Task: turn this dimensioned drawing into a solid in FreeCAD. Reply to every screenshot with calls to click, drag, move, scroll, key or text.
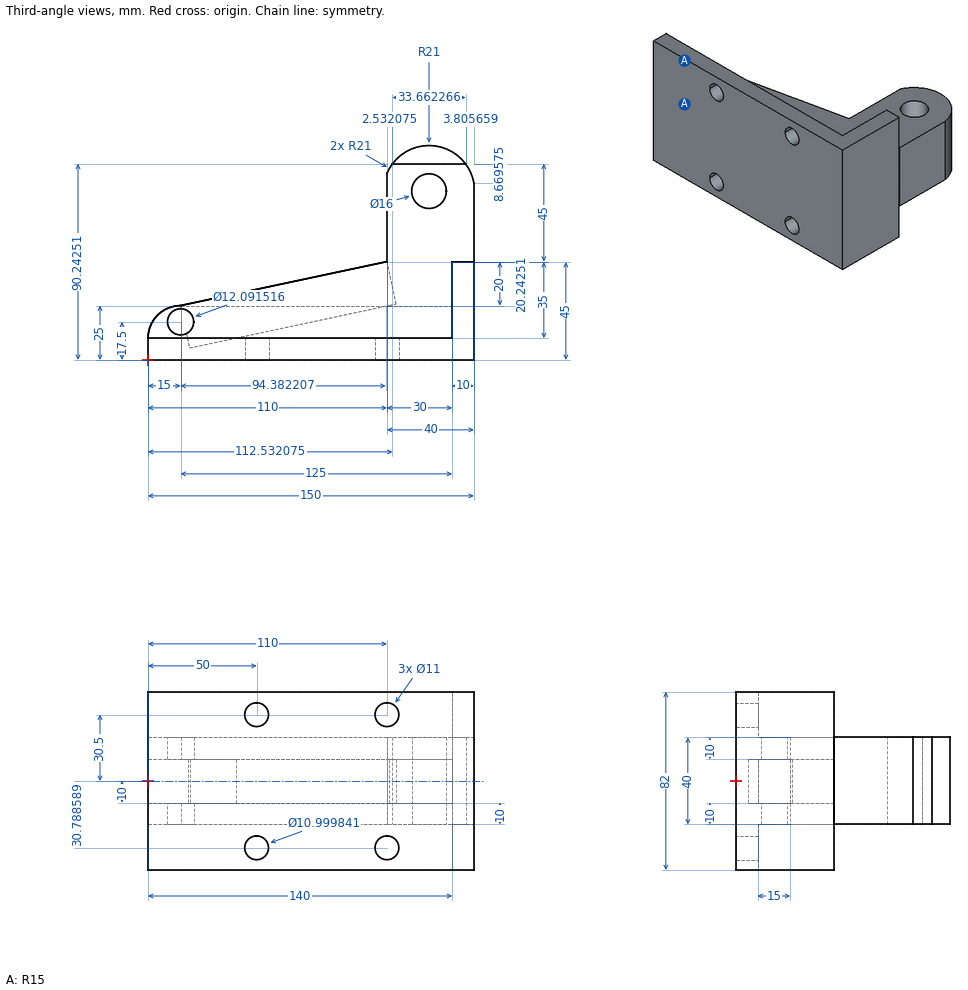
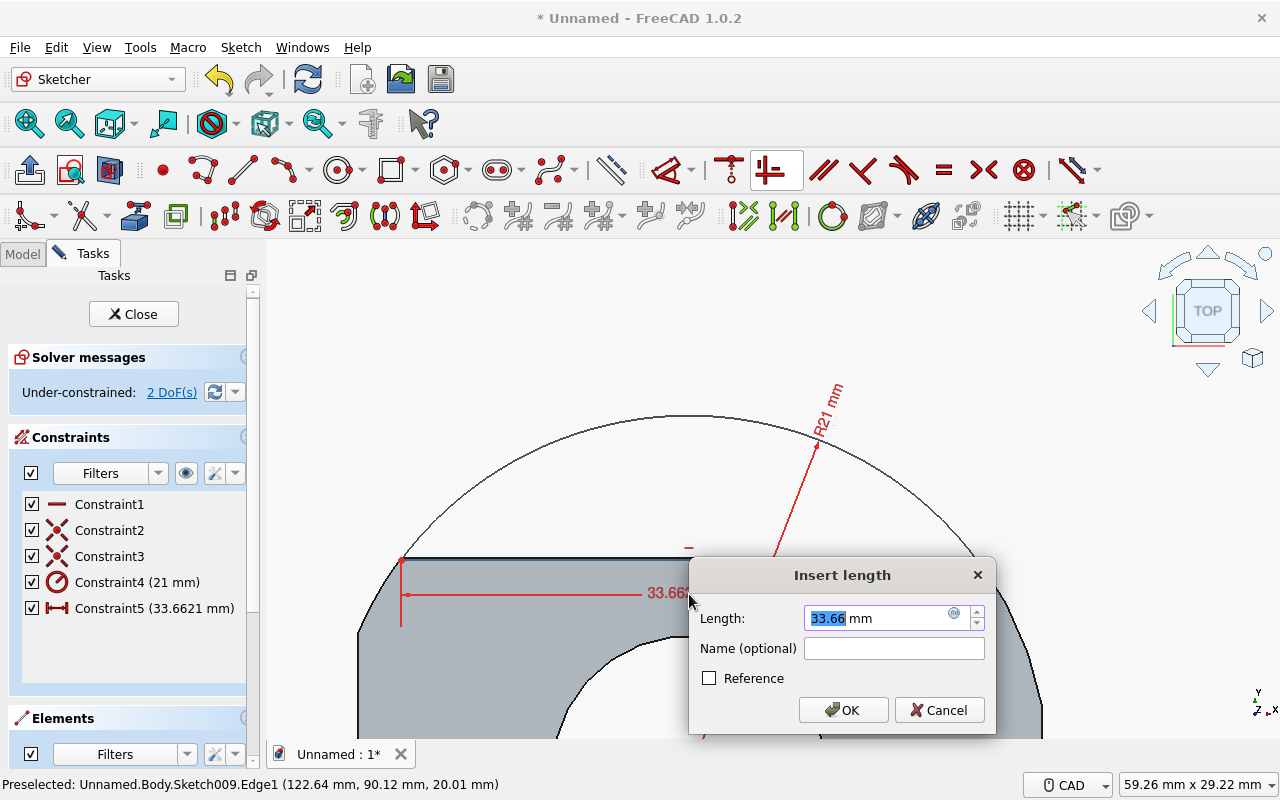
text(33.662266)
key(Return)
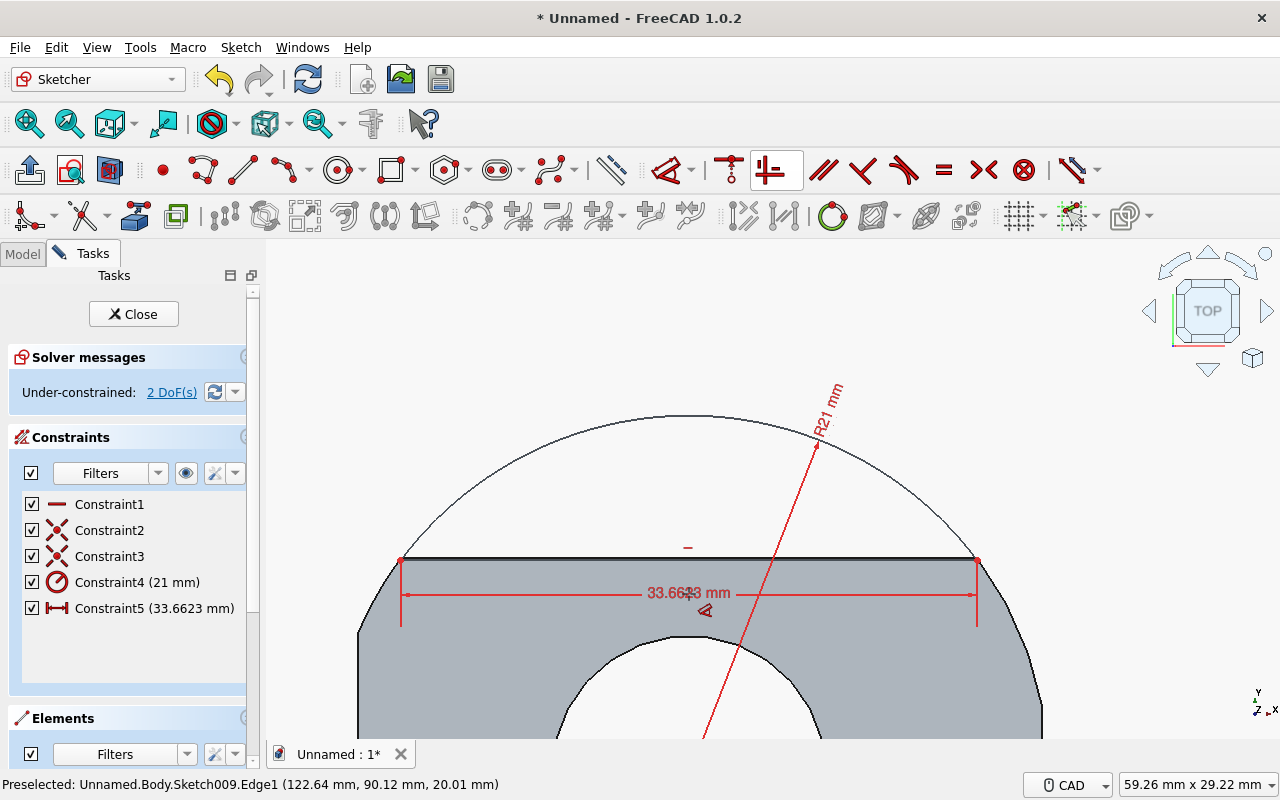
click(401, 560)
click(435, 636)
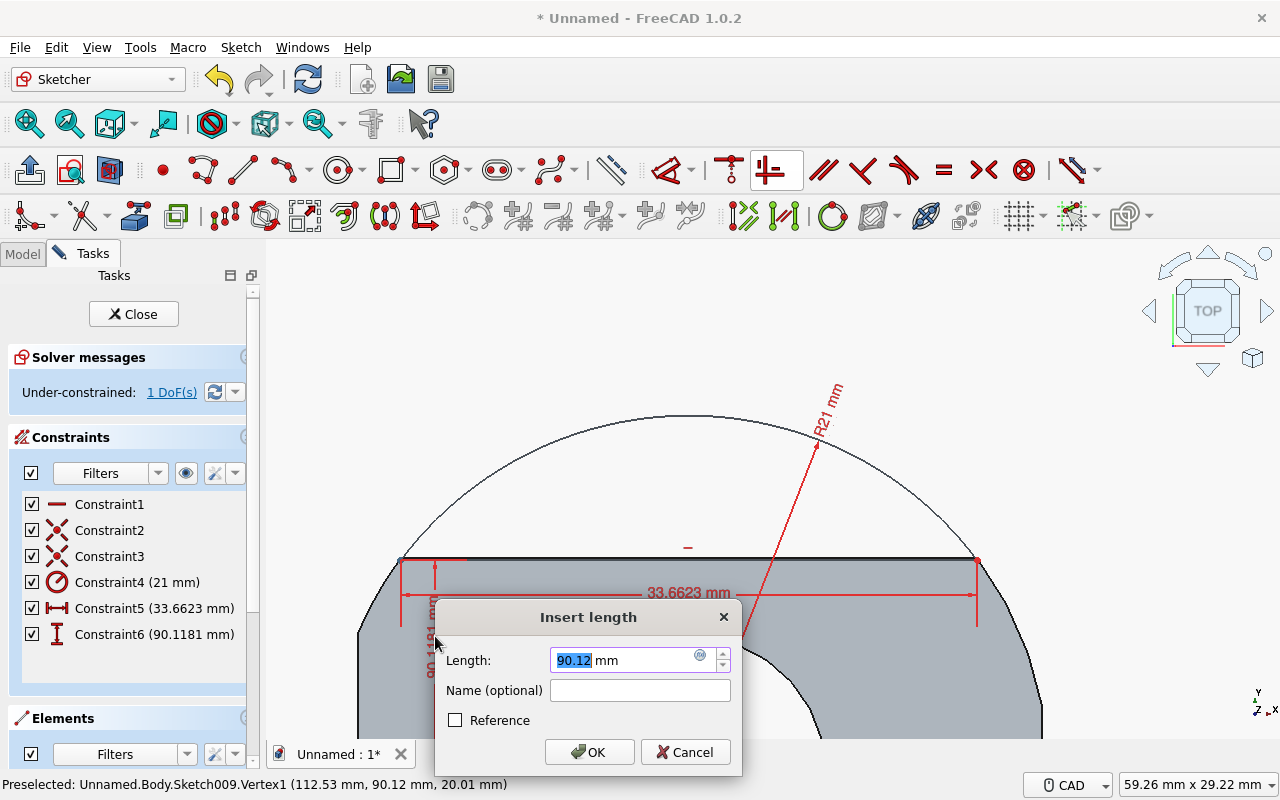
text(90.24251)
key(Return)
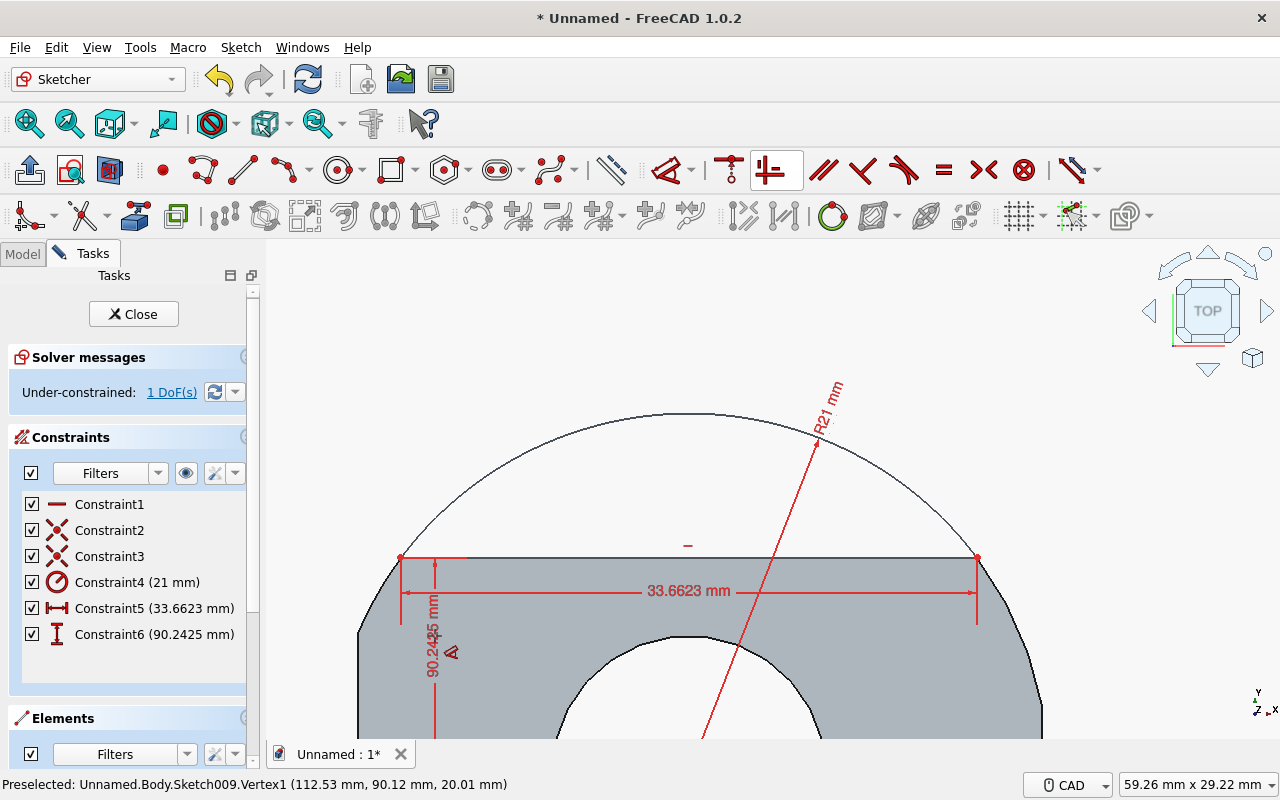
click(401, 558)
click(347, 524)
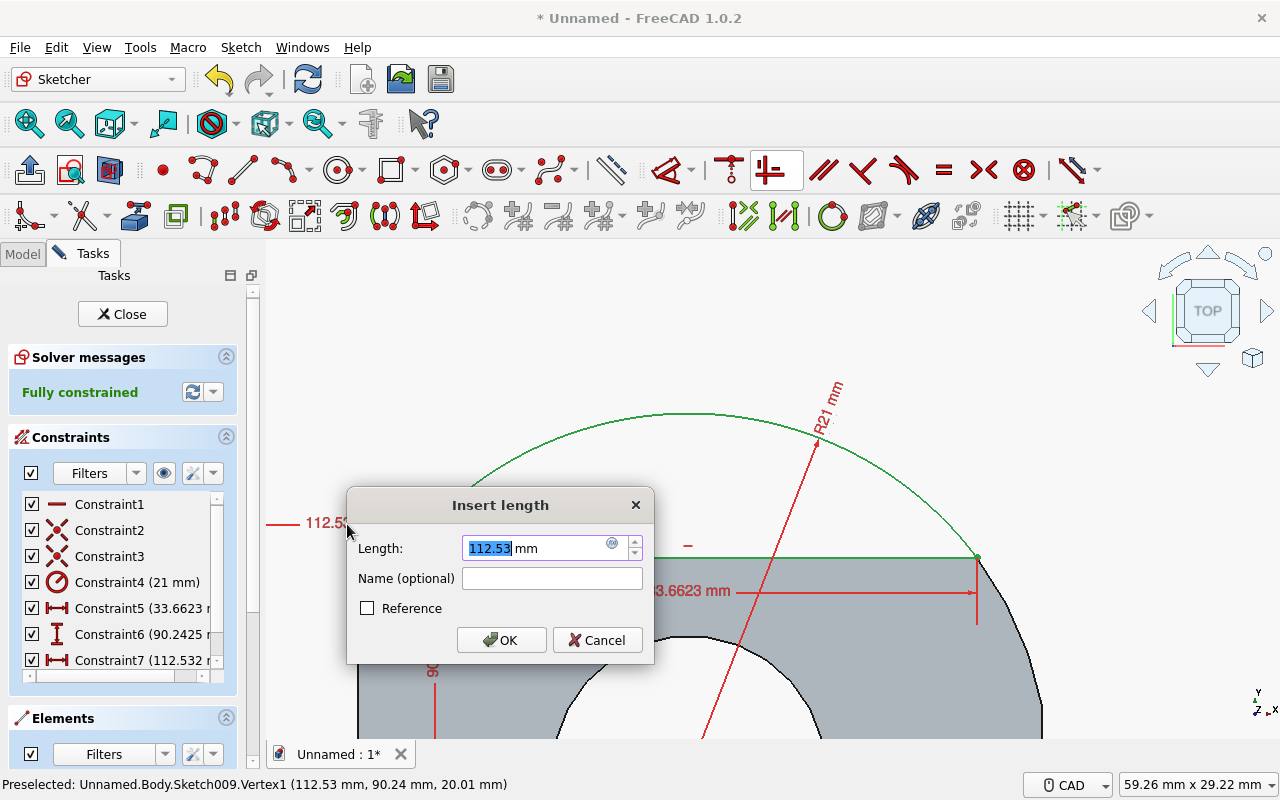
text(112.532075)
key(Return)
key(Escape)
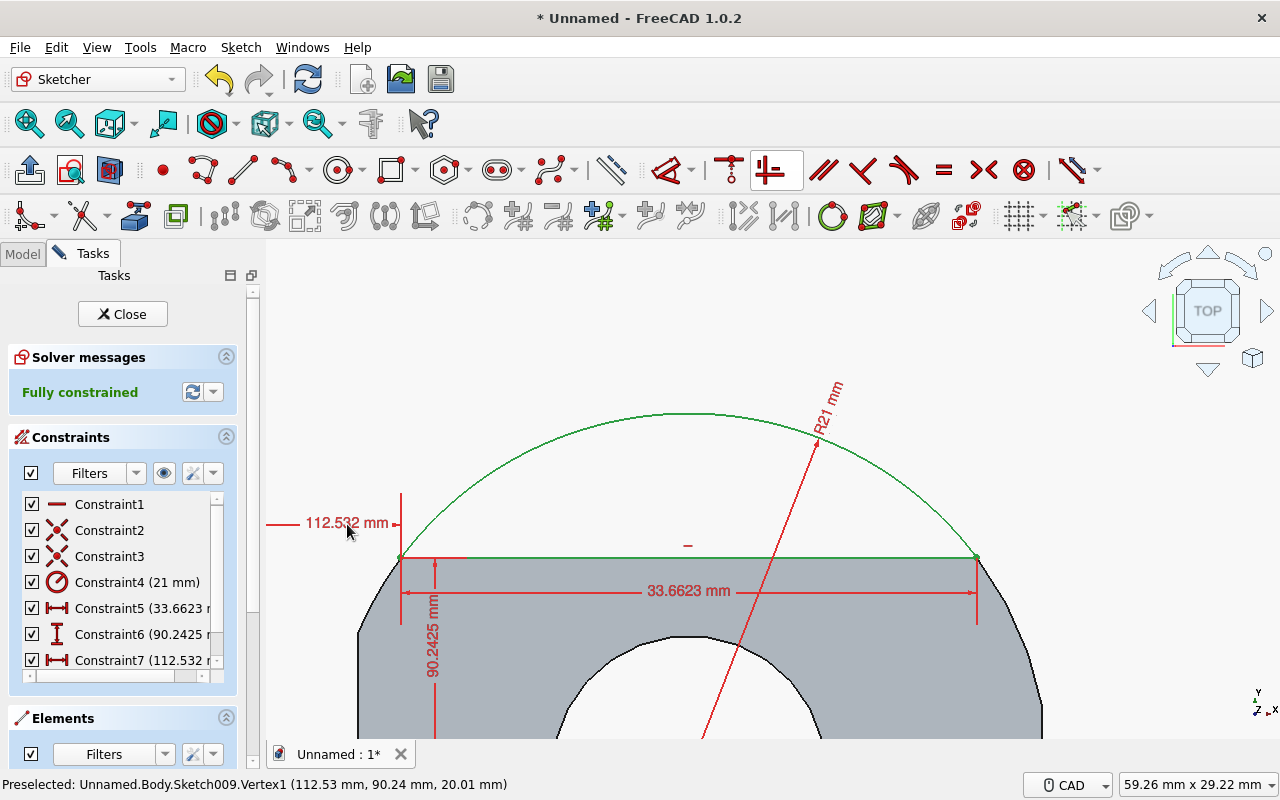
click(123, 314)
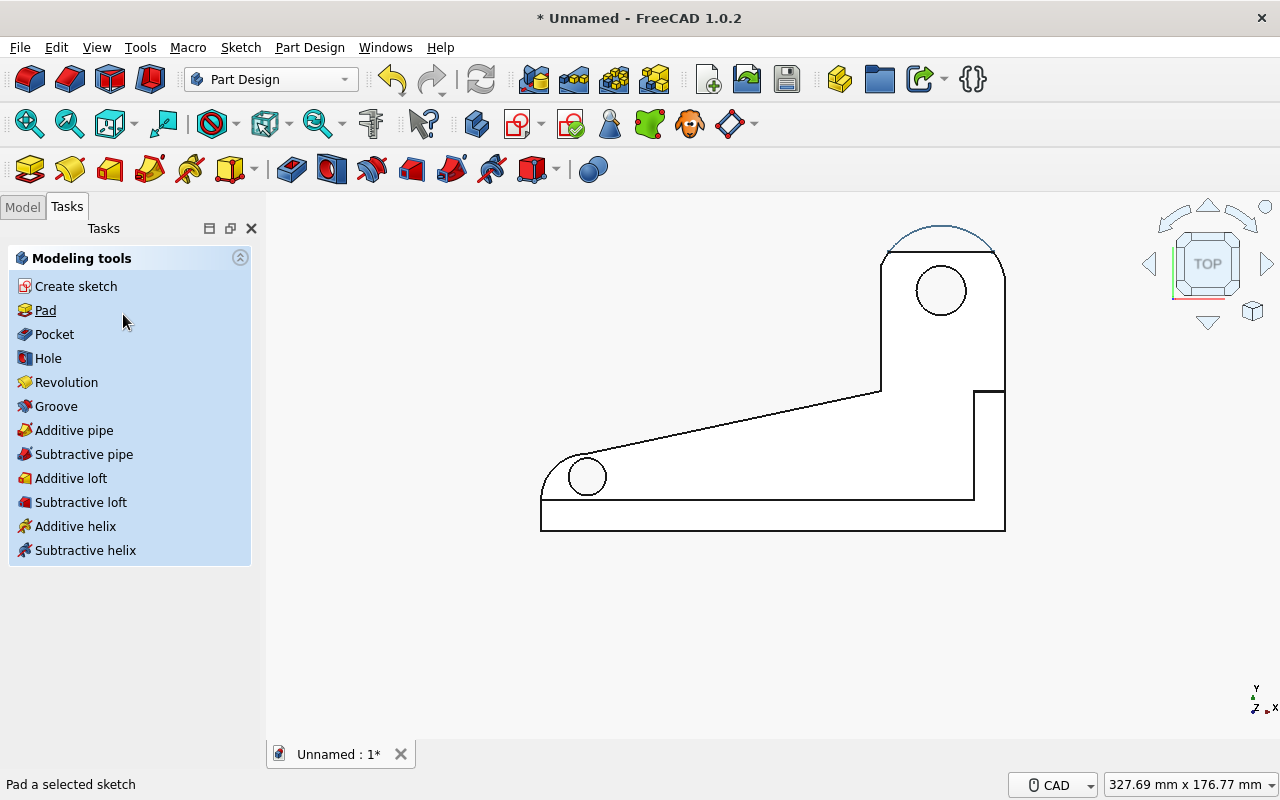
click(30, 170)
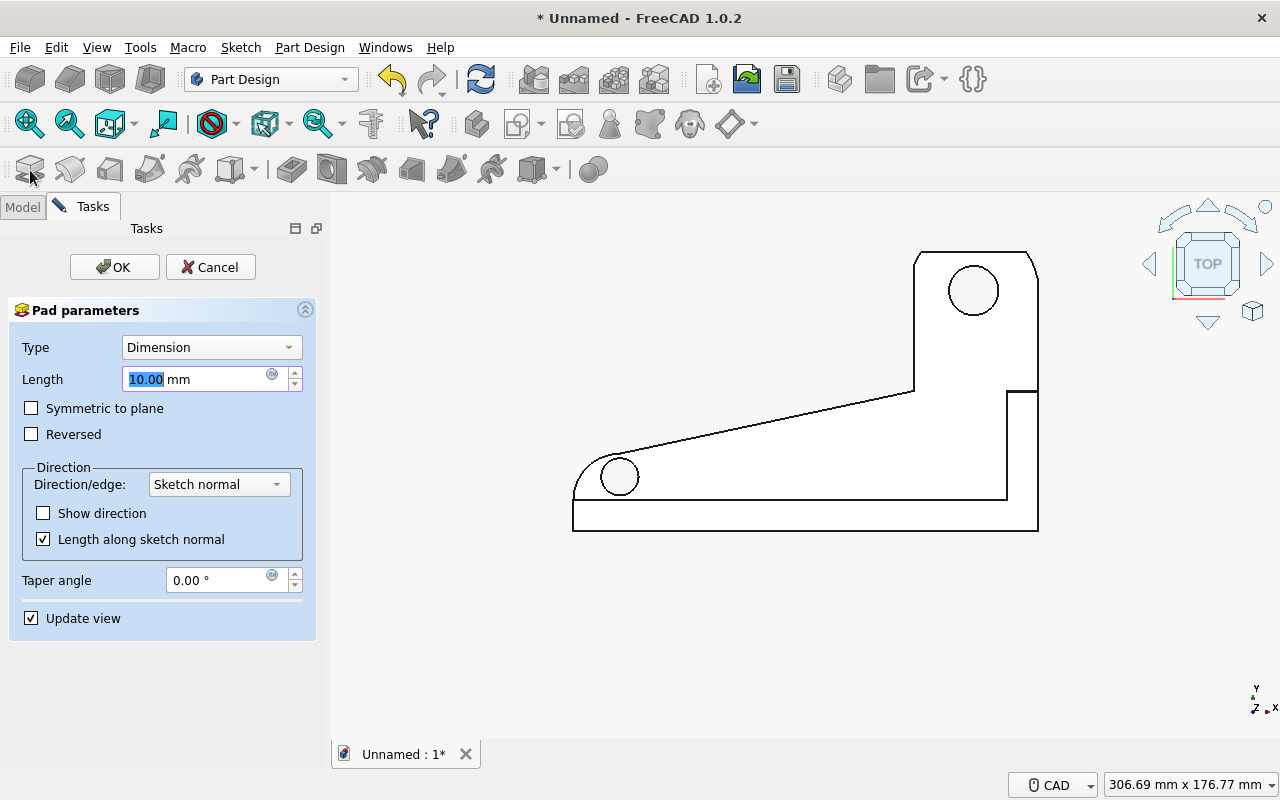
text(40)
key(Tab)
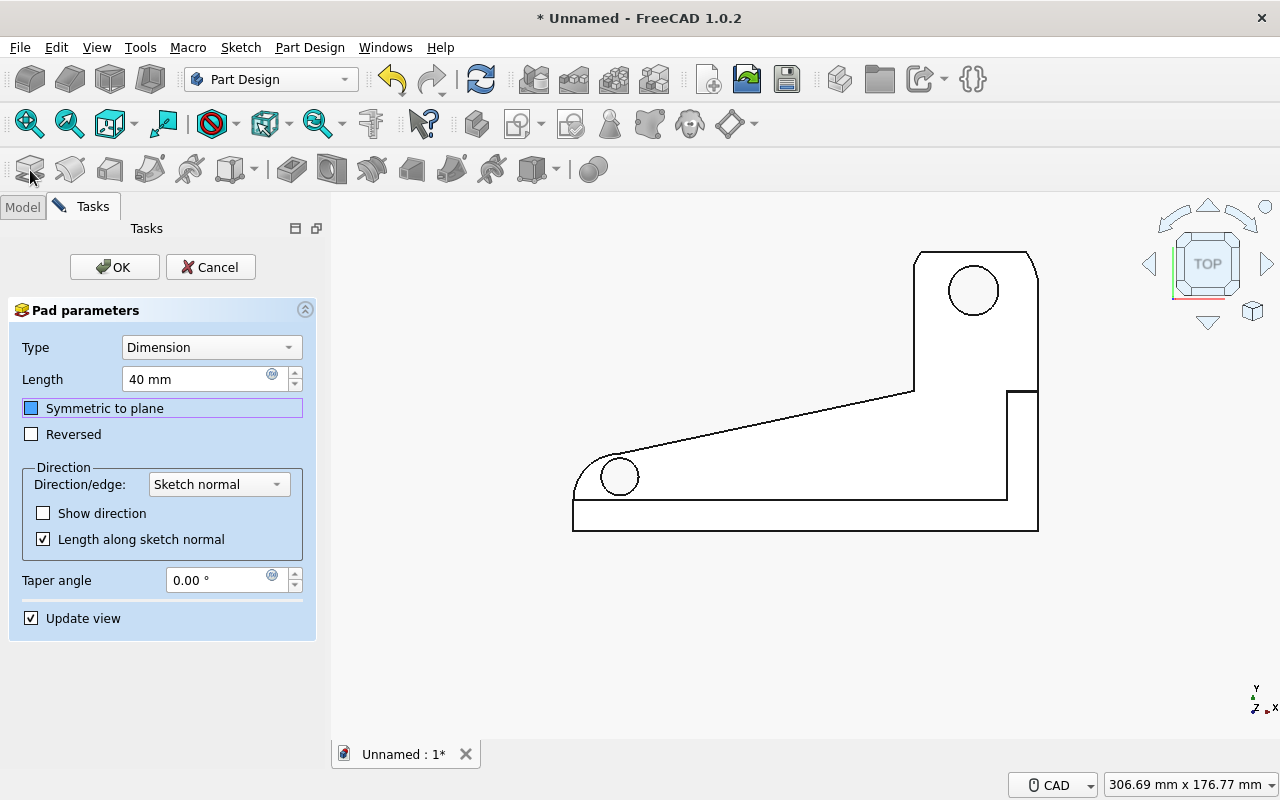
click(30, 434)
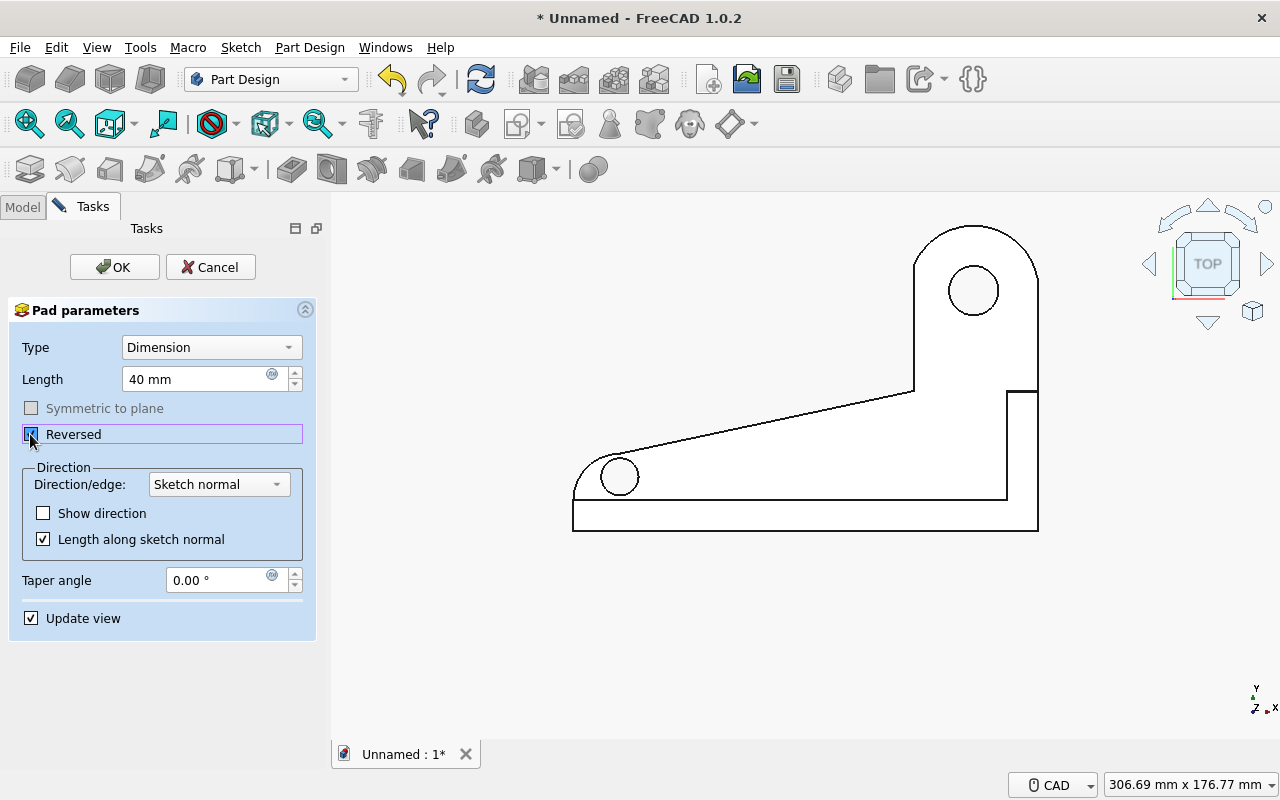
click(115, 267)